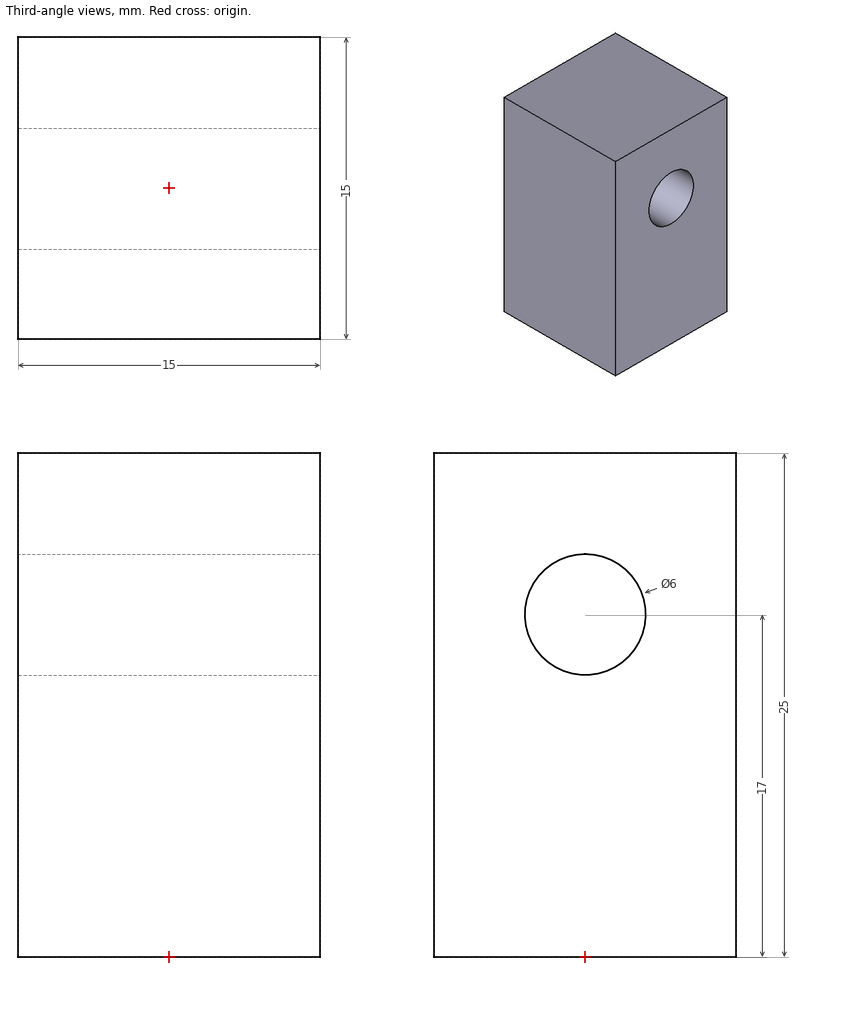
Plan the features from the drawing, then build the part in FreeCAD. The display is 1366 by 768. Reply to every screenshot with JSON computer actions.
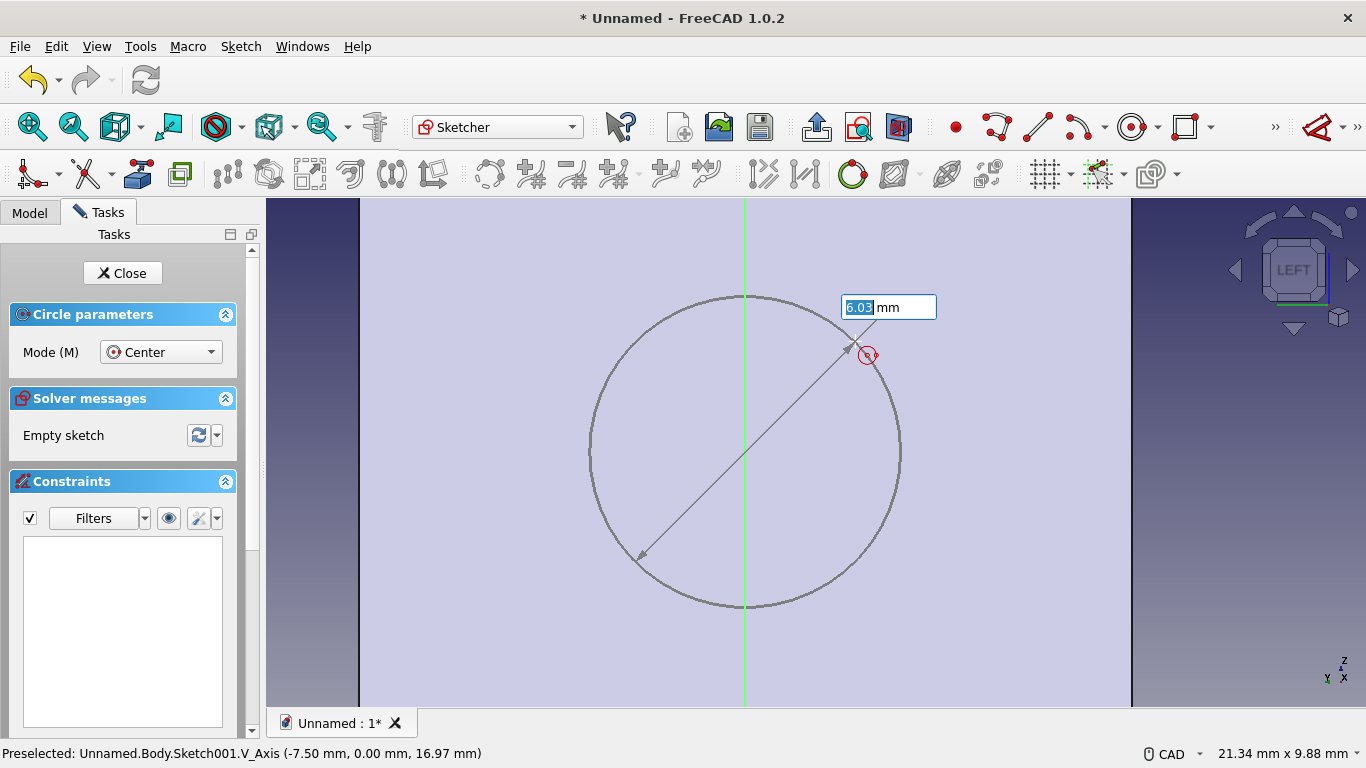
{"action": "type", "text": "6"}
{"action": "key", "text": "Return"}
{"action": "key", "text": "Escape"}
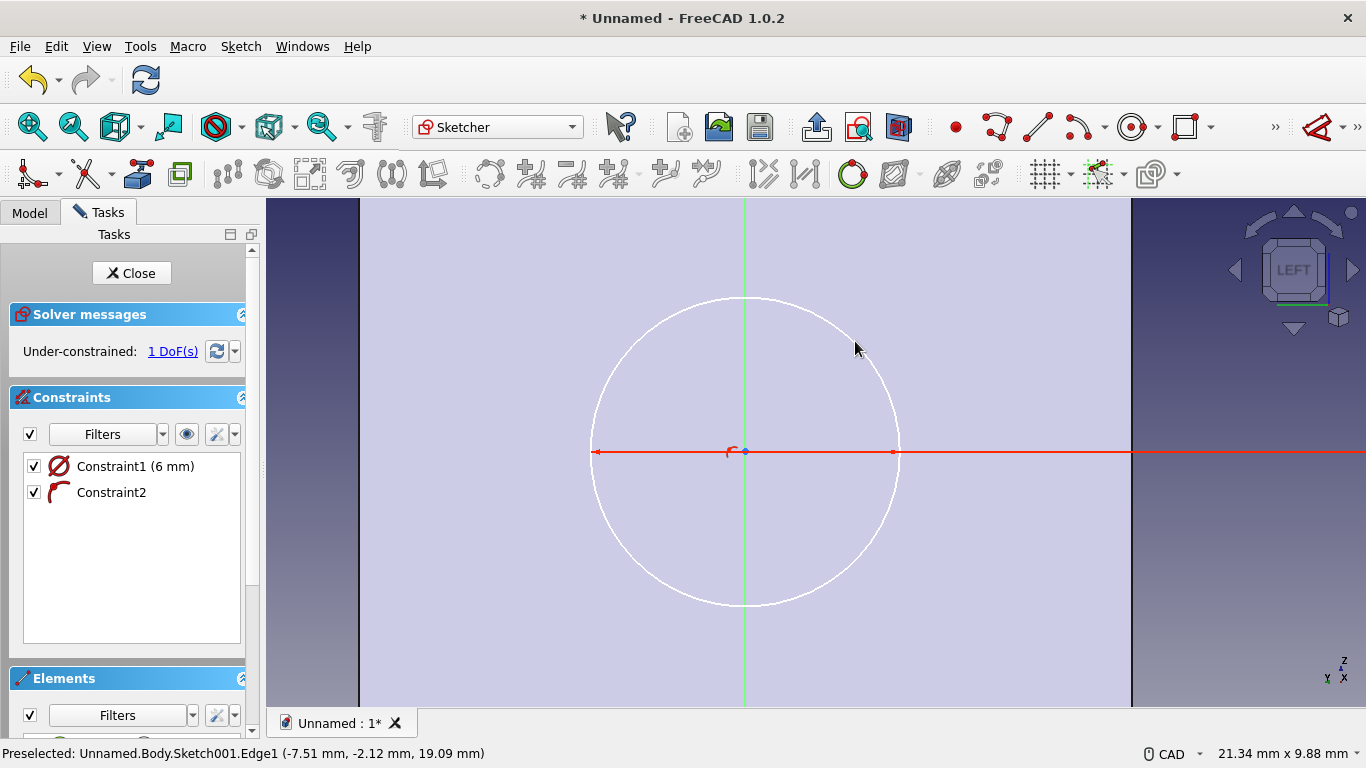
{"action": "key", "text": "d"}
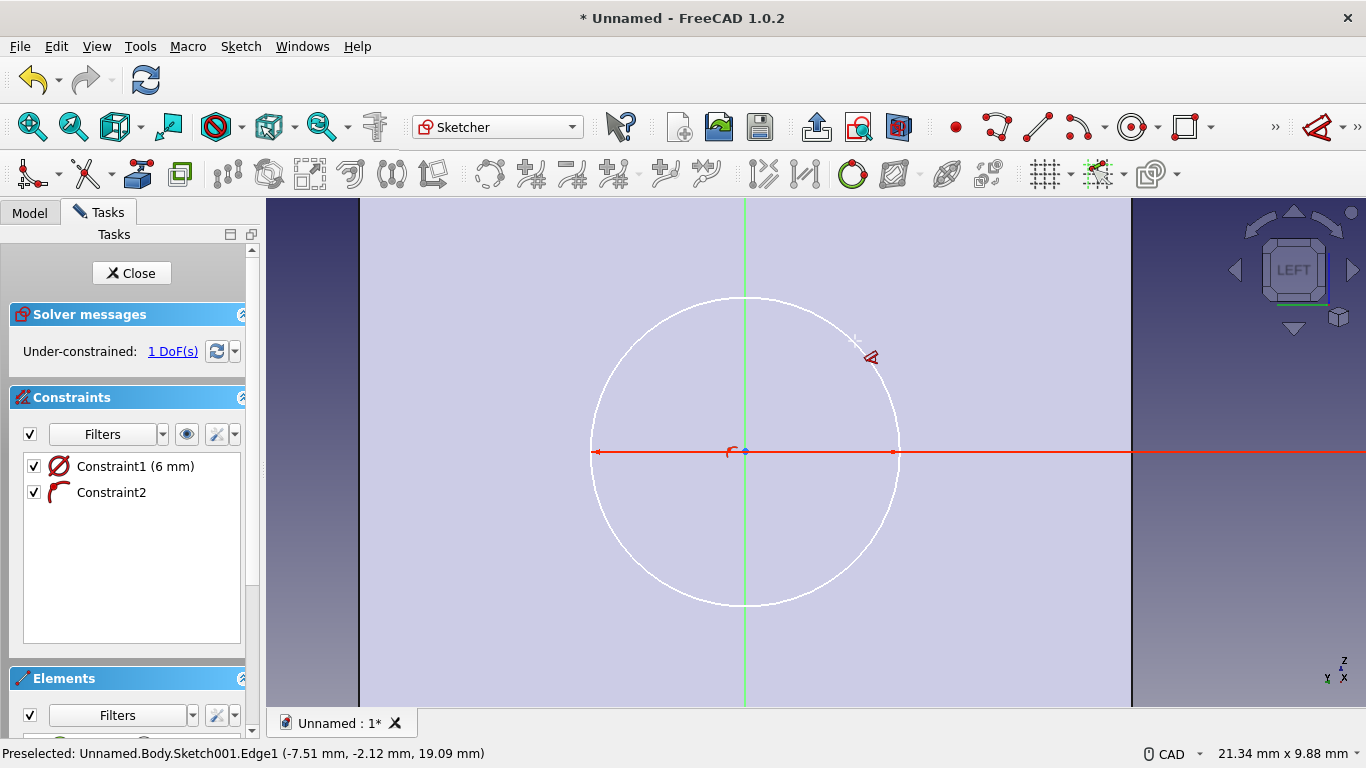
{"action": "left_click", "coordinate": [745, 452]}
{"action": "left_click", "coordinate": [779, 565]}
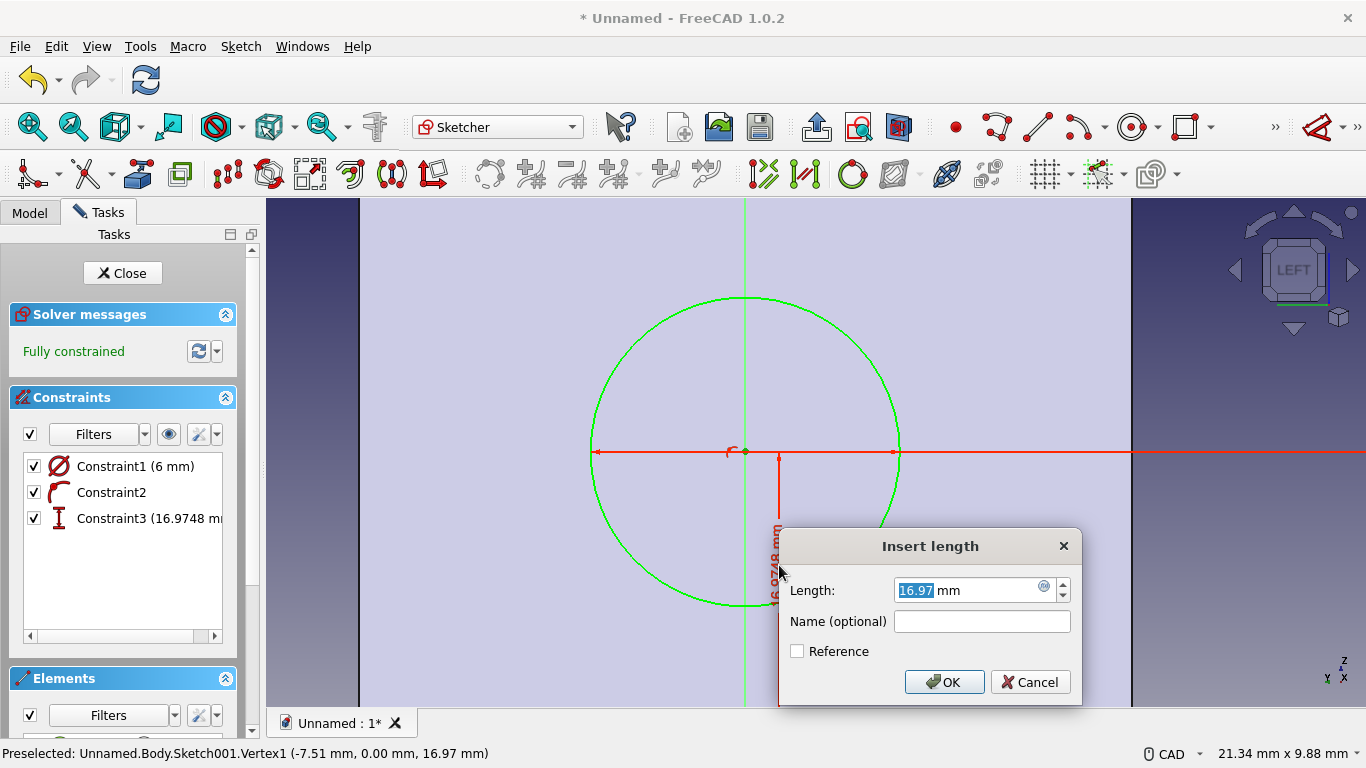
{"action": "type", "text": "17"}
{"action": "key", "text": "Return"}
{"action": "key", "text": "Escape"}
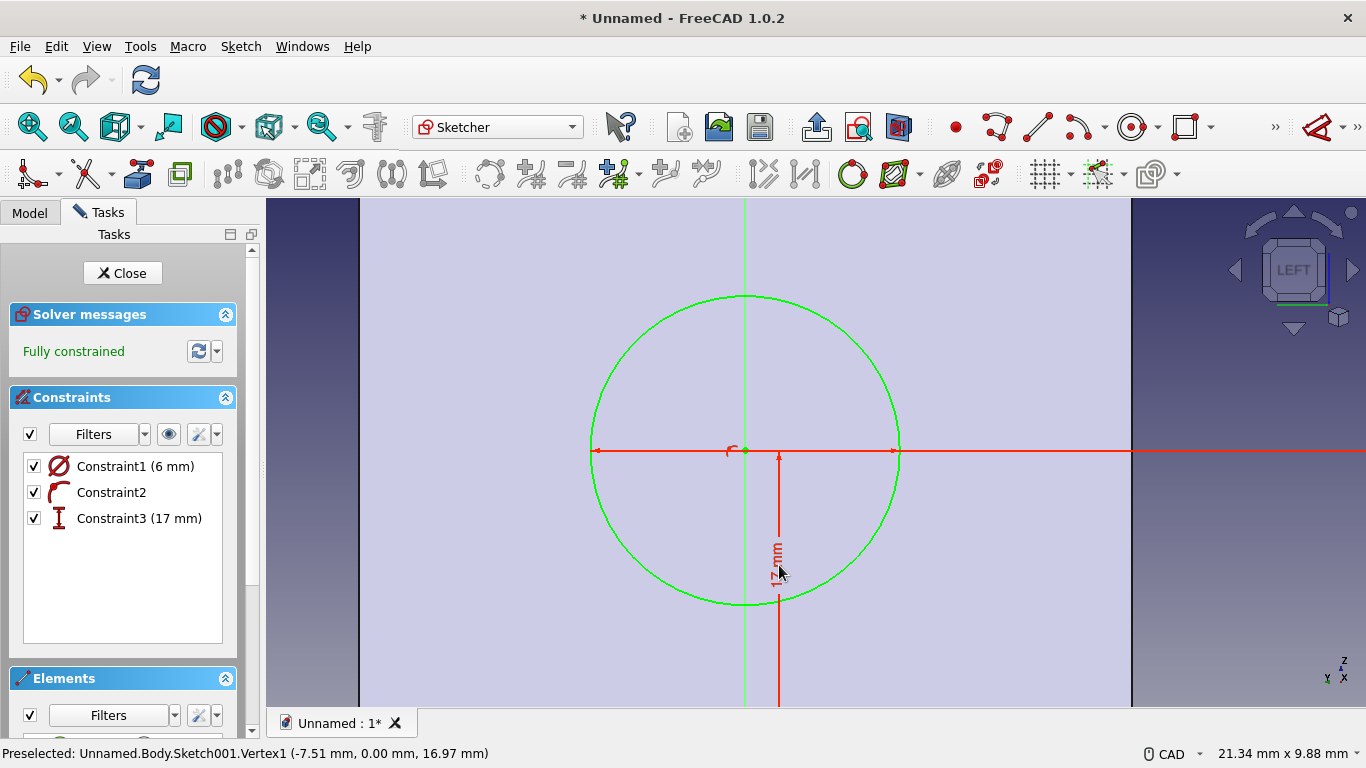
{"action": "left_click", "coordinate": [123, 273]}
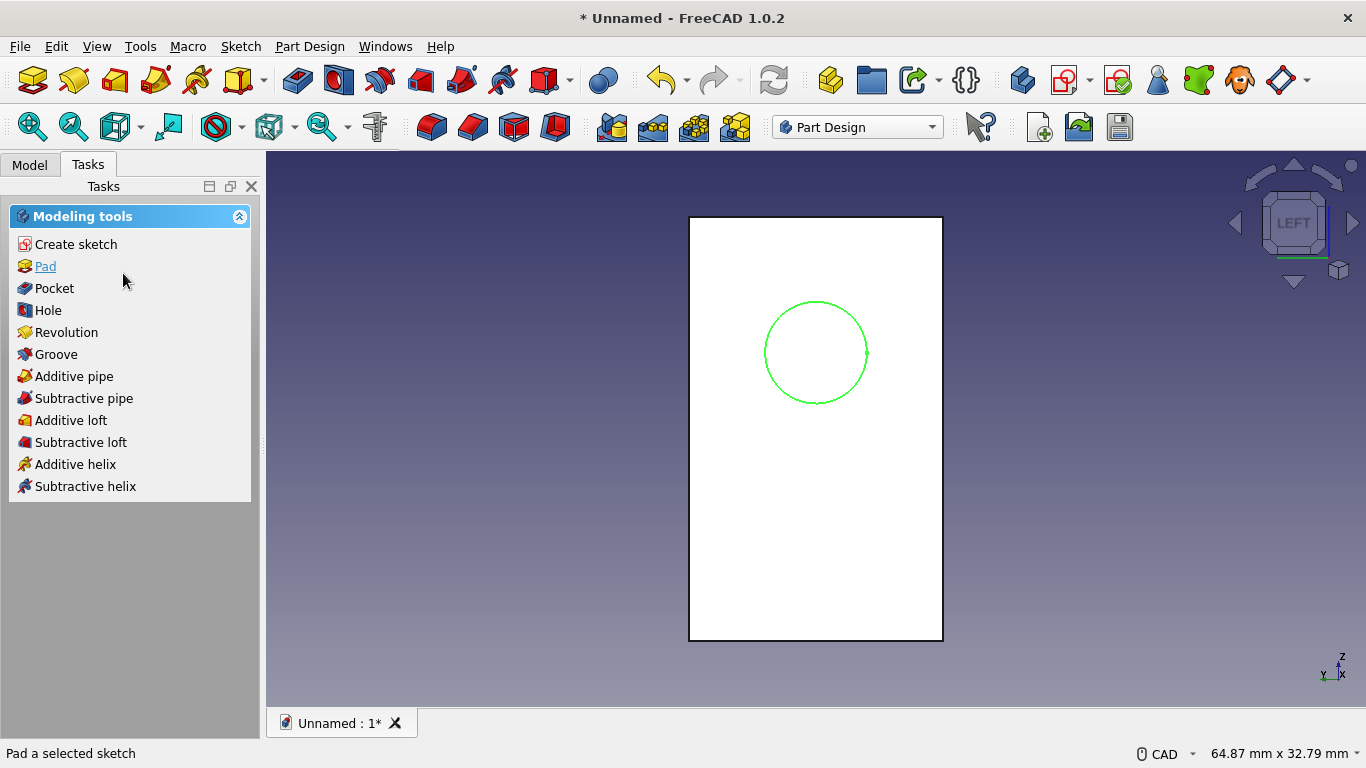
{"action": "left_click", "coordinate": [298, 80]}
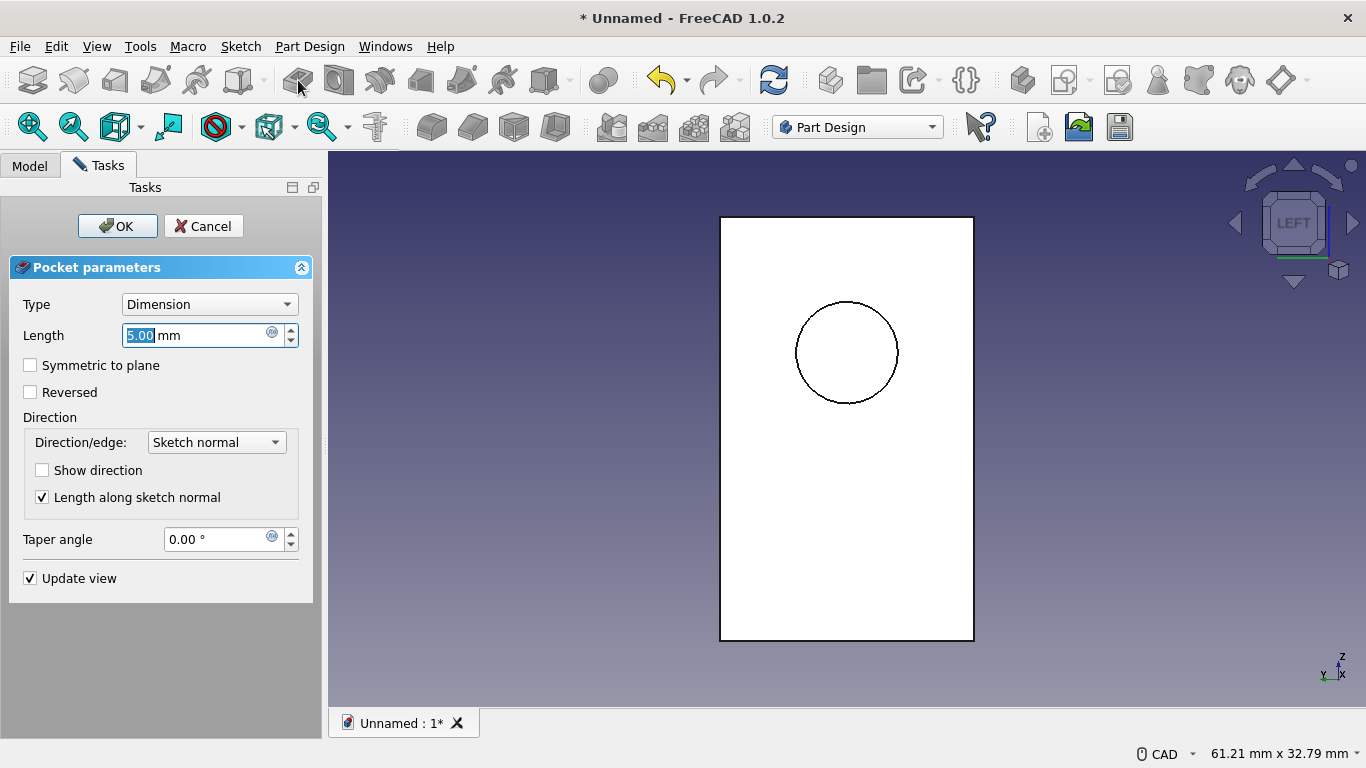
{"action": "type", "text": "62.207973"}
{"action": "key", "text": "Tab"}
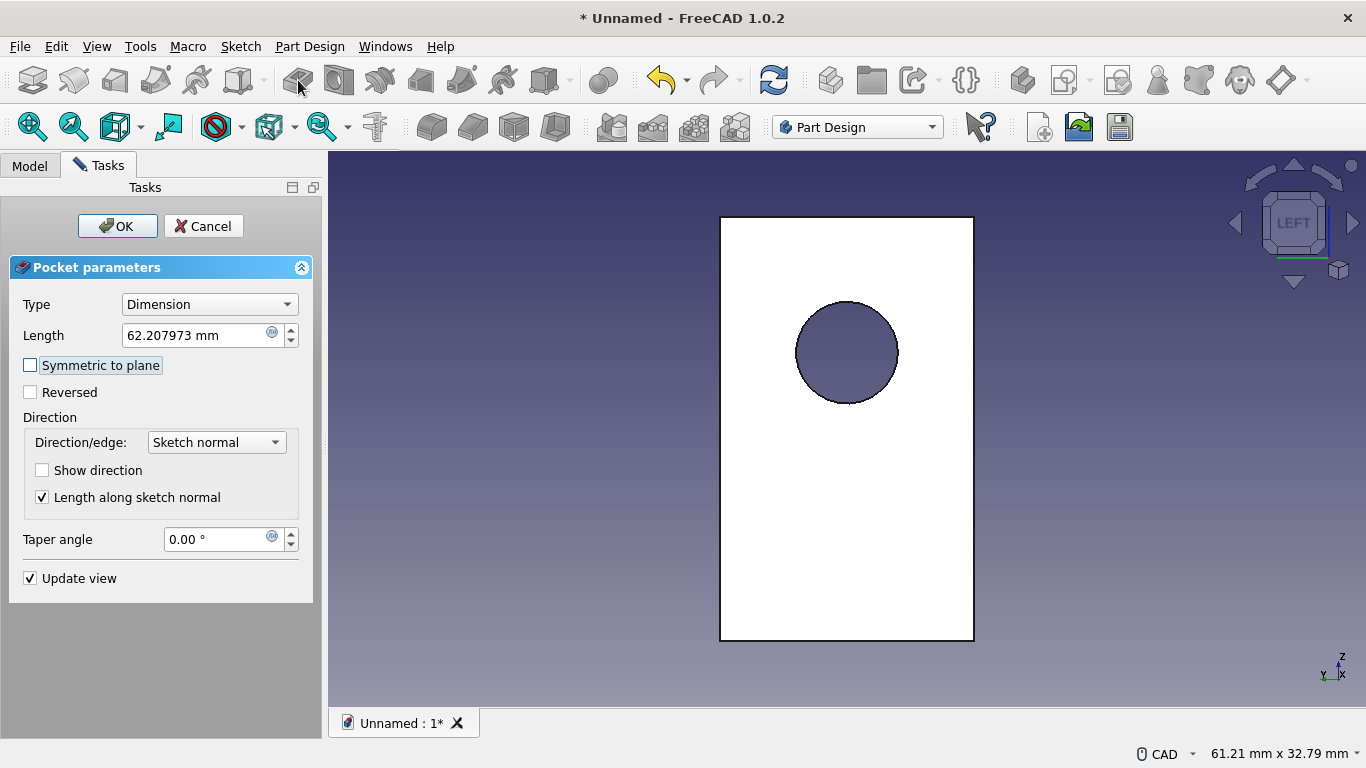
{"action": "left_click", "coordinate": [31, 365]}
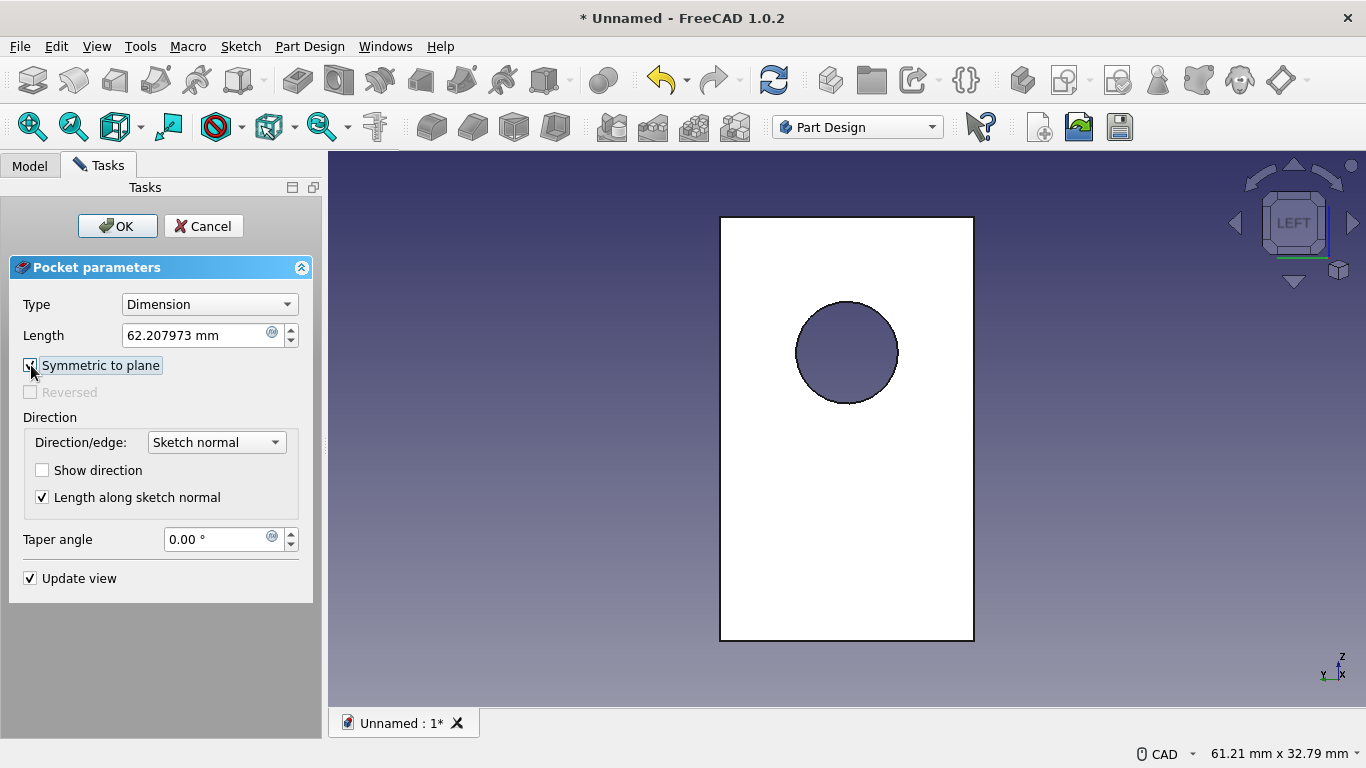
{"action": "left_click", "coordinate": [118, 226]}